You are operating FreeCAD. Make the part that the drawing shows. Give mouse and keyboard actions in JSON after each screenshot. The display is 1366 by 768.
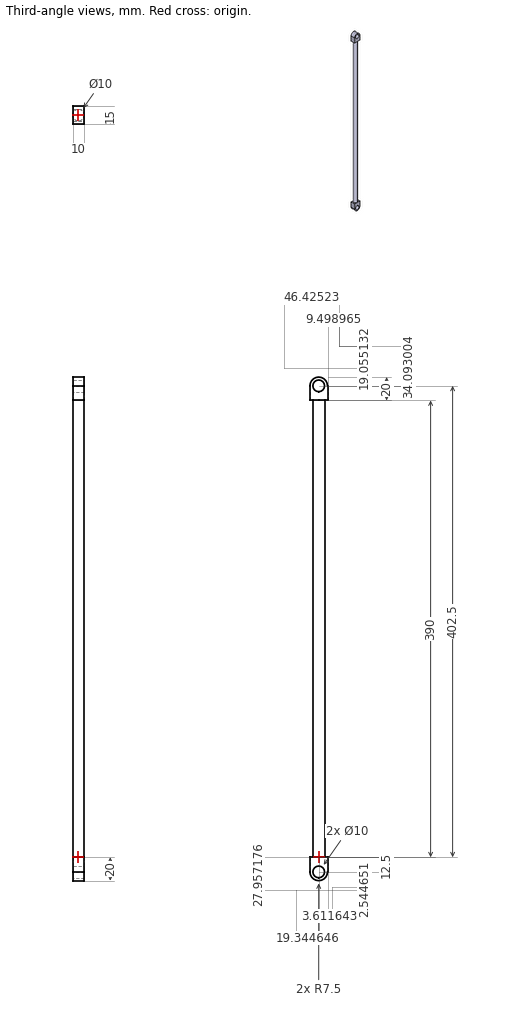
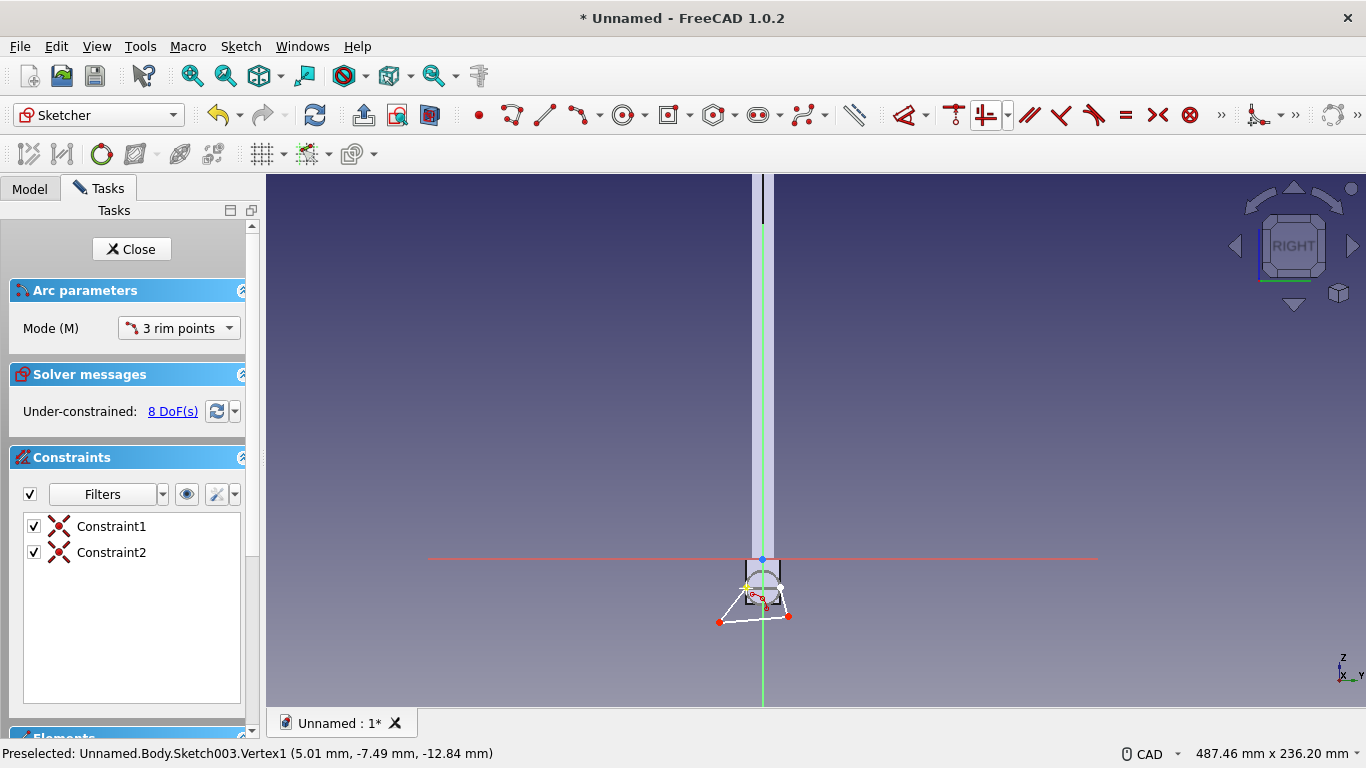
{"action": "scroll", "coordinate": [753, 601], "scroll_direction": "up", "scroll_amount": 3}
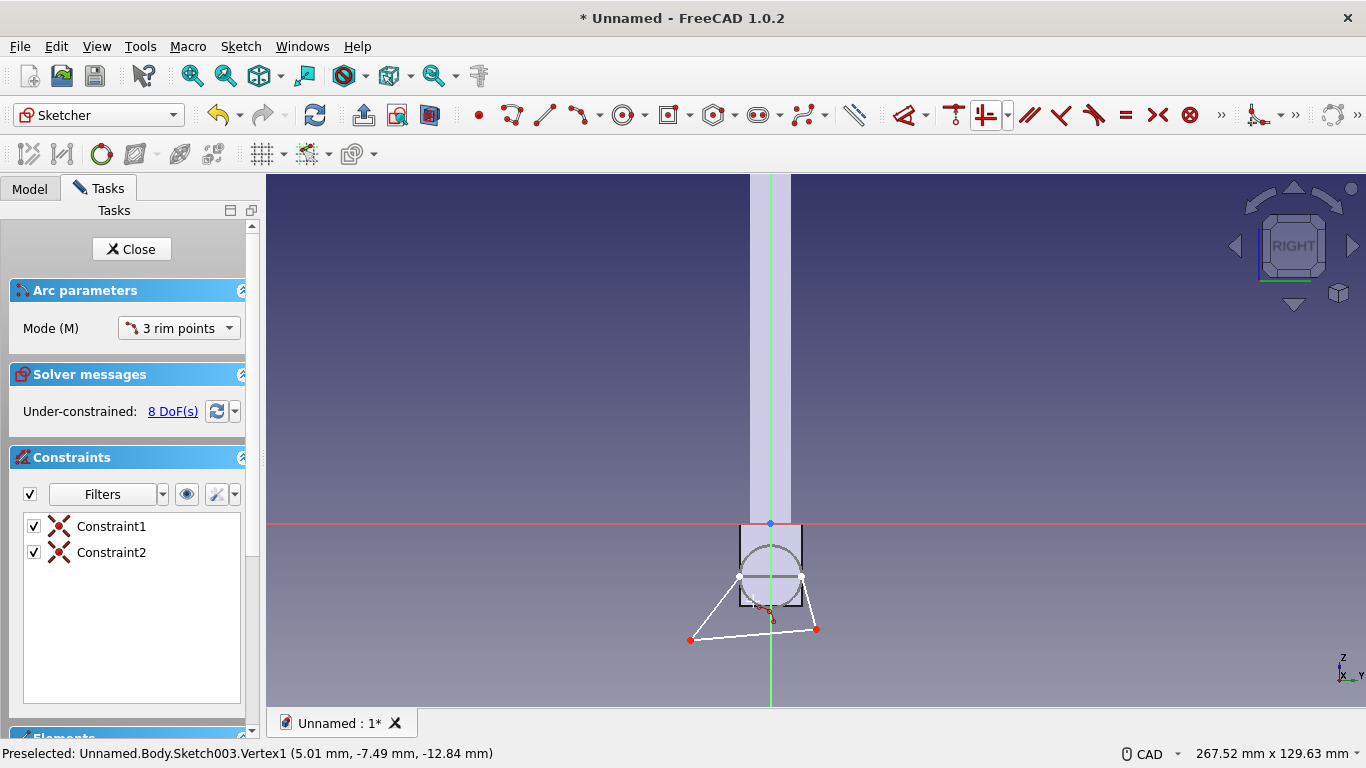
{"action": "left_click", "coordinate": [753, 600]}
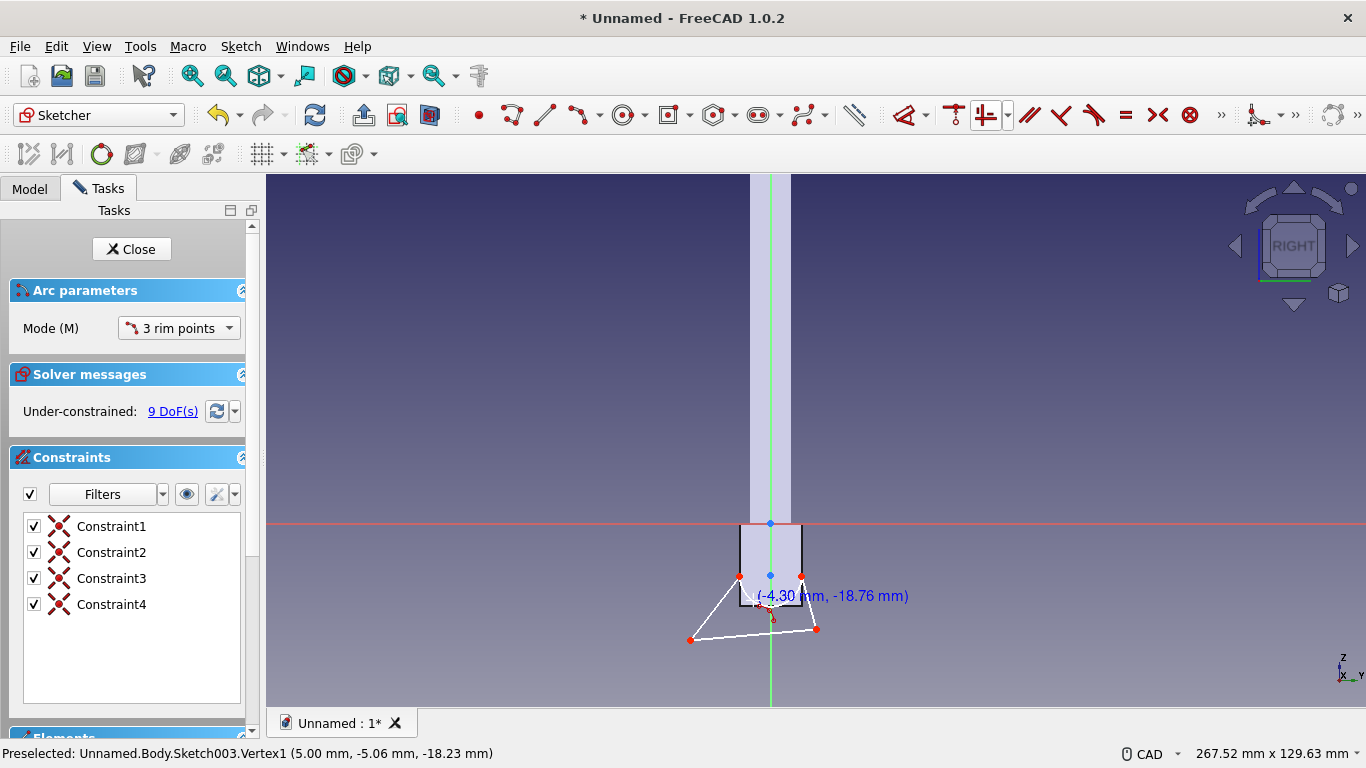
{"action": "left_click", "coordinate": [512, 116]}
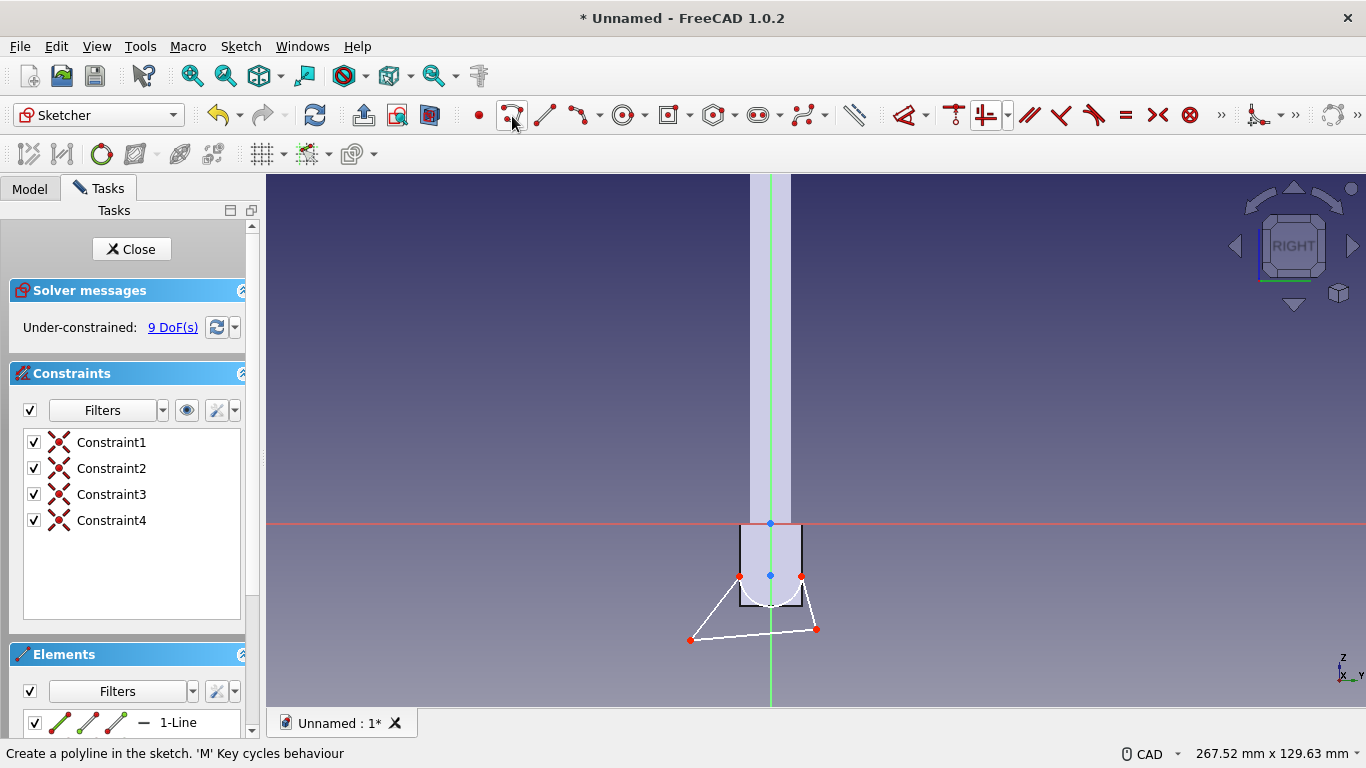
{"action": "scroll", "coordinate": [748, 590], "scroll_direction": "down", "scroll_amount": 9}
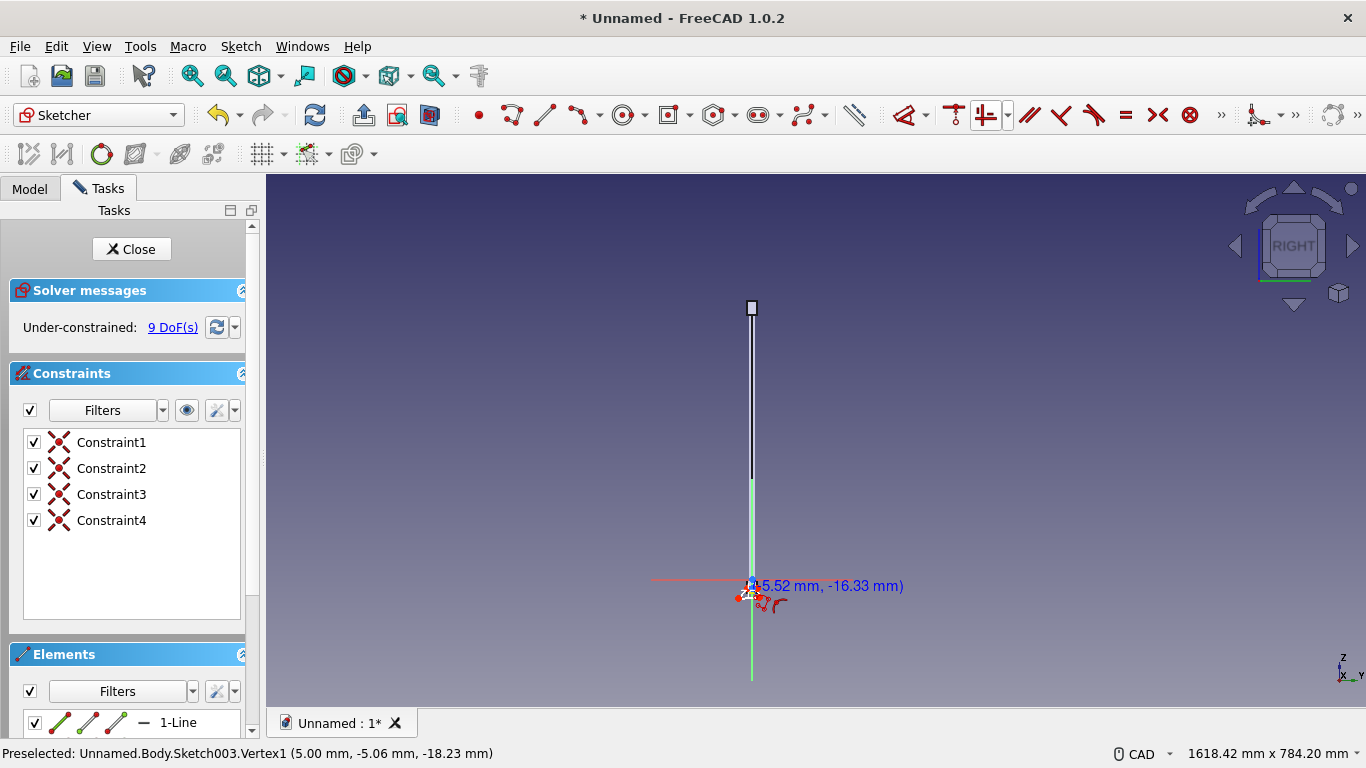
{"action": "scroll", "coordinate": [757, 306], "scroll_direction": "up", "scroll_amount": 6}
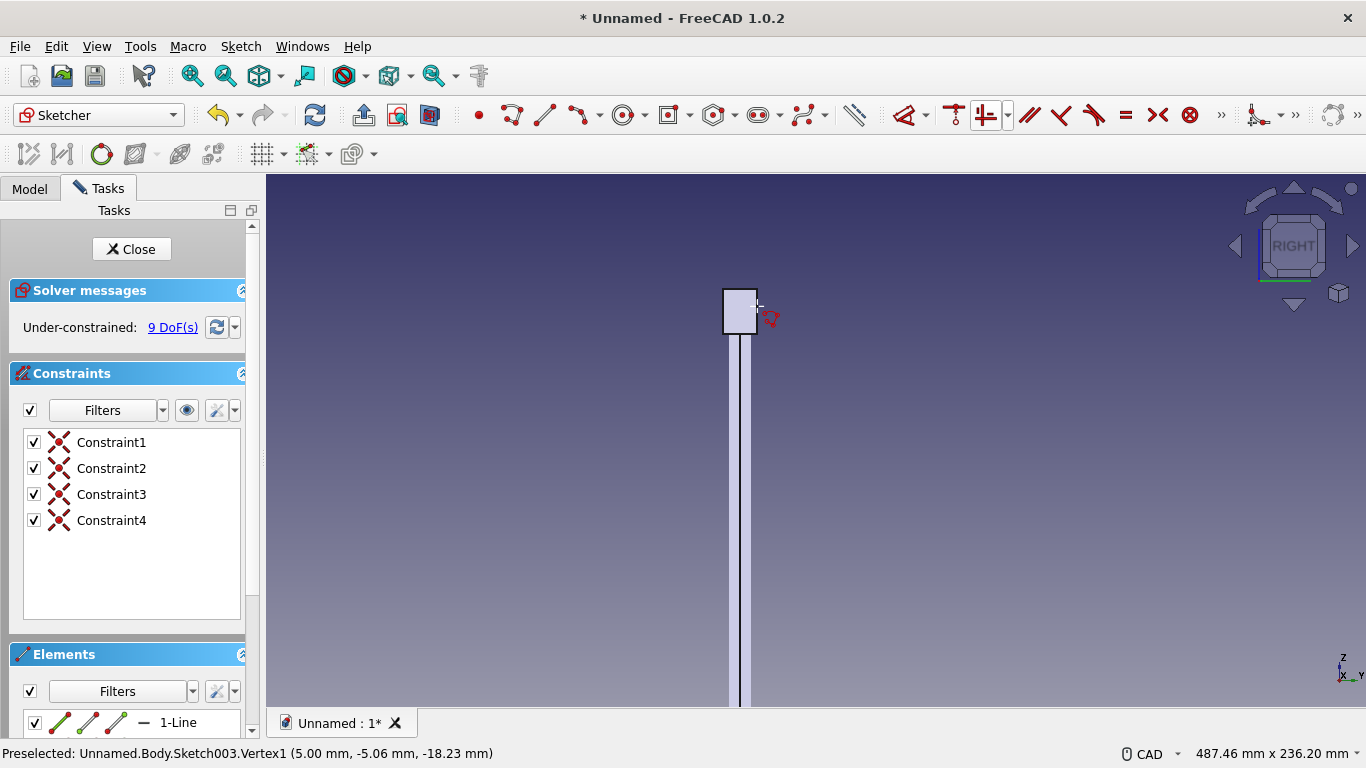
{"action": "left_click", "coordinate": [757, 306]}
{"action": "left_click", "coordinate": [778, 229]}
{"action": "left_click", "coordinate": [673, 272]}
{"action": "left_click", "coordinate": [723, 306]}
{"action": "right_click", "coordinate": [723, 306]}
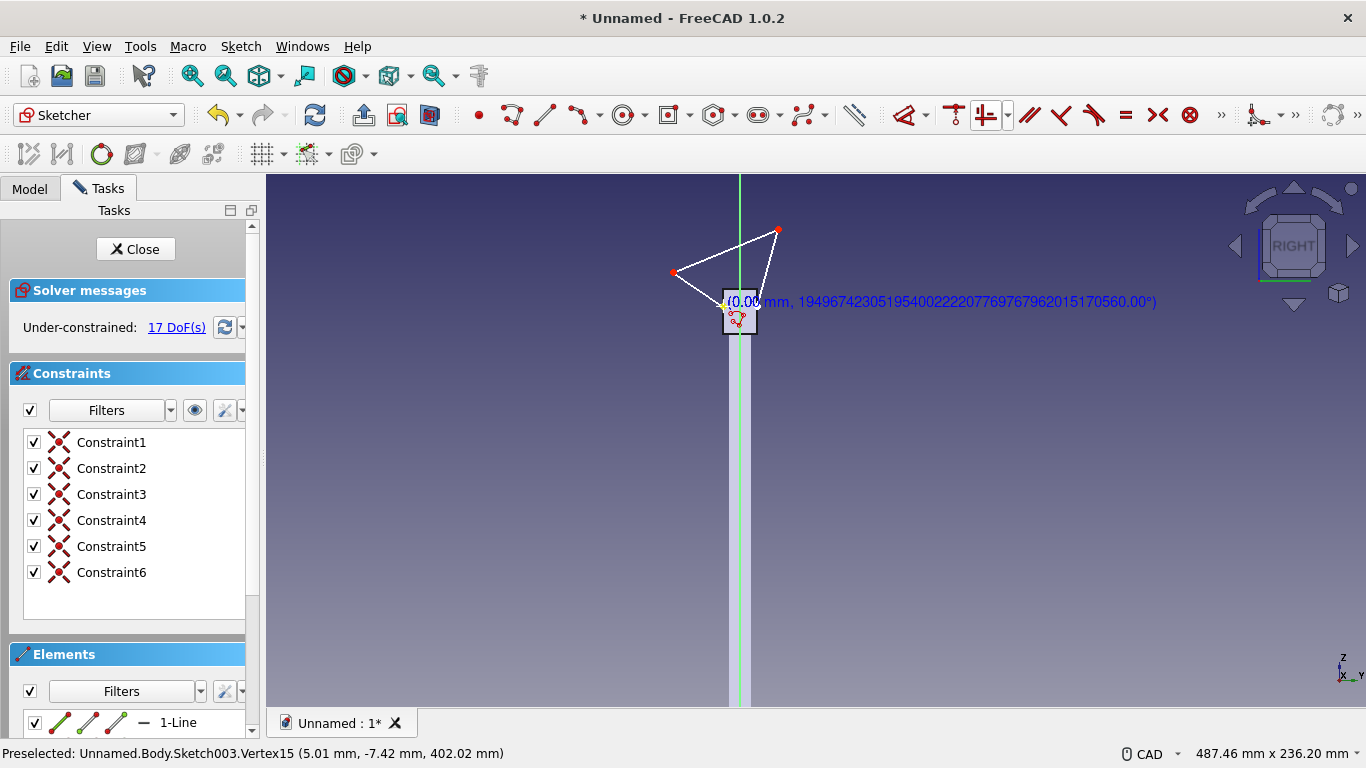
{"action": "left_click", "coordinate": [578, 116]}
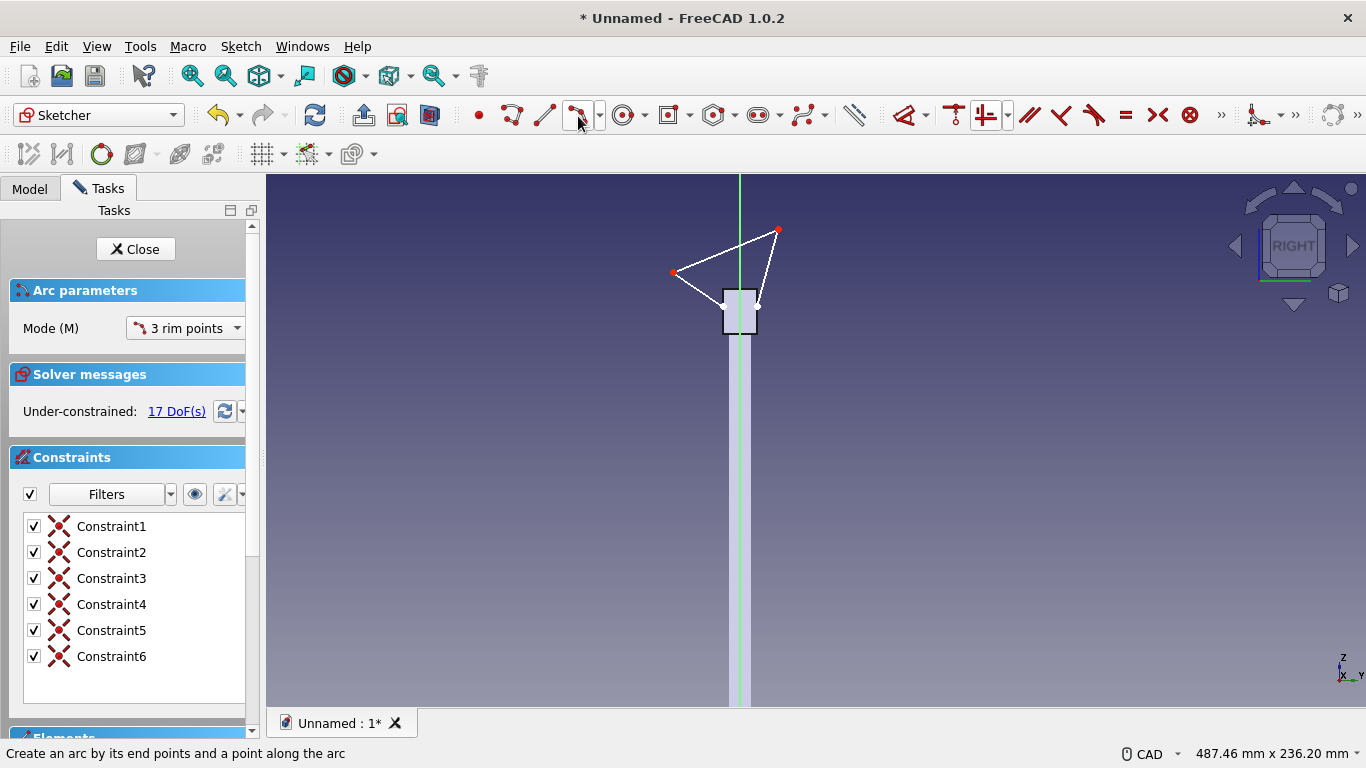
{"action": "left_click", "coordinate": [723, 307]}
{"action": "left_click", "coordinate": [757, 307]}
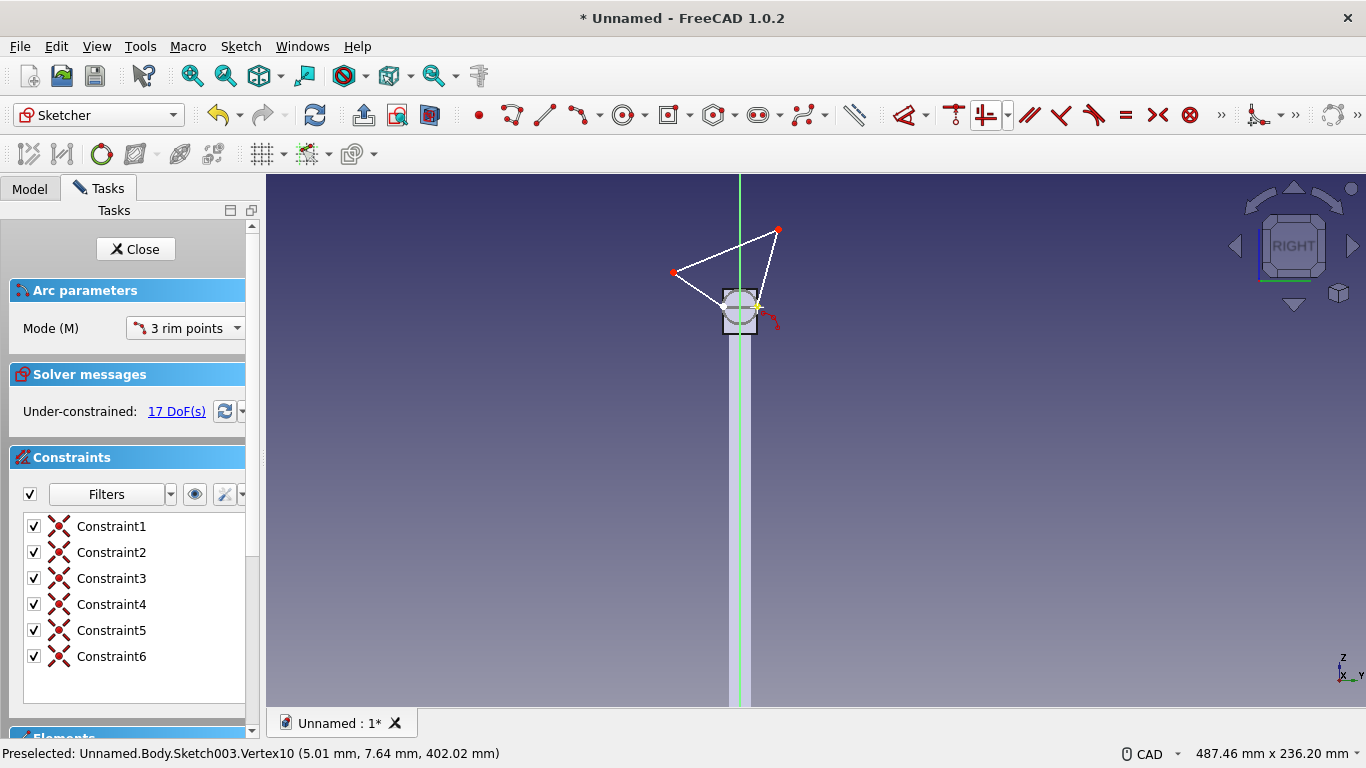
{"action": "scroll", "coordinate": [750, 292], "scroll_direction": "up", "scroll_amount": 3}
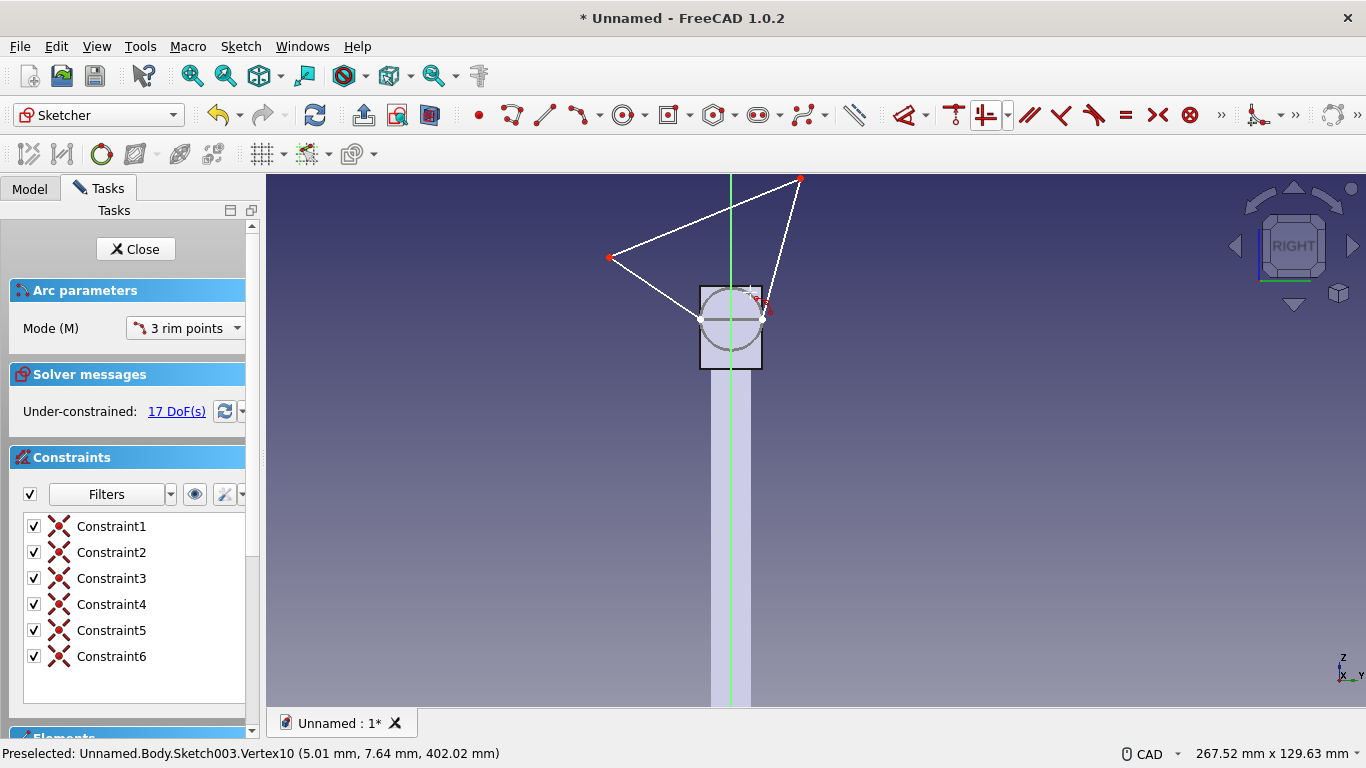
{"action": "left_click", "coordinate": [749, 292]}